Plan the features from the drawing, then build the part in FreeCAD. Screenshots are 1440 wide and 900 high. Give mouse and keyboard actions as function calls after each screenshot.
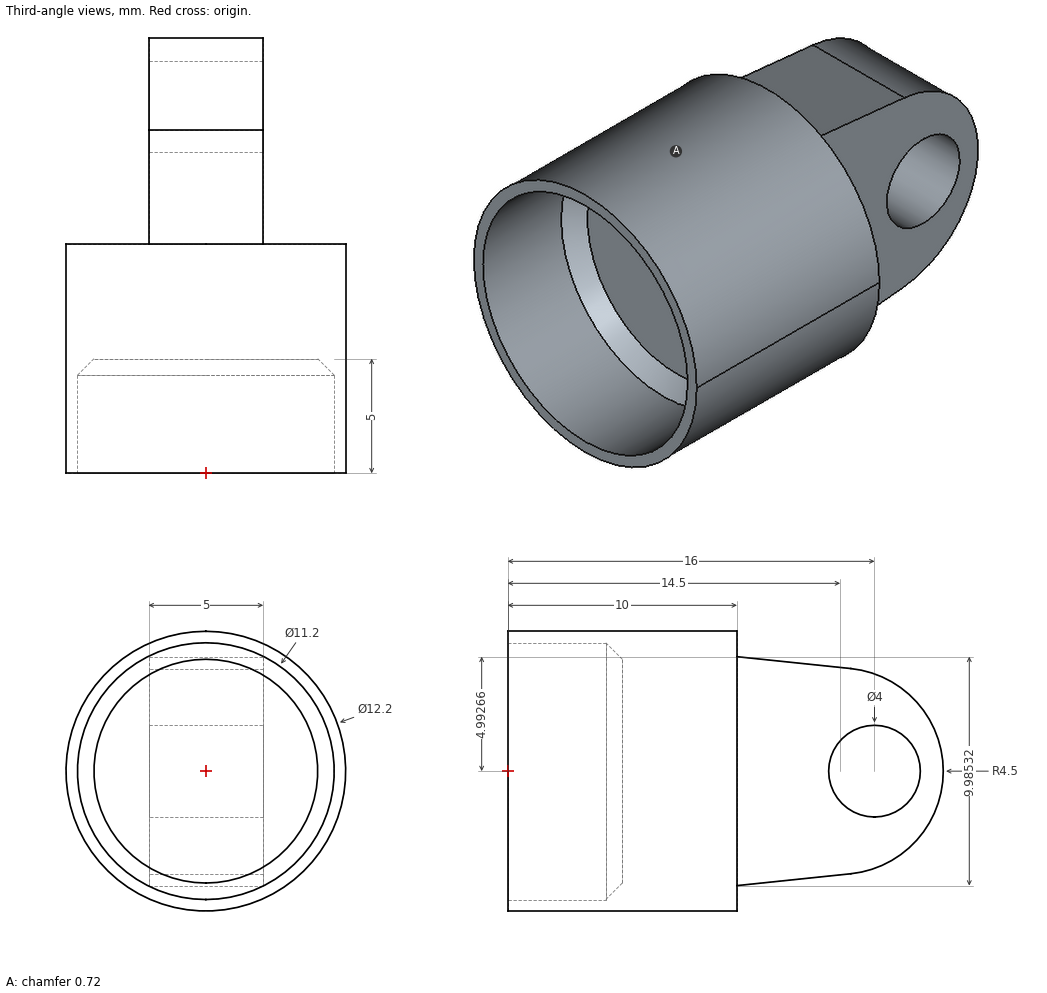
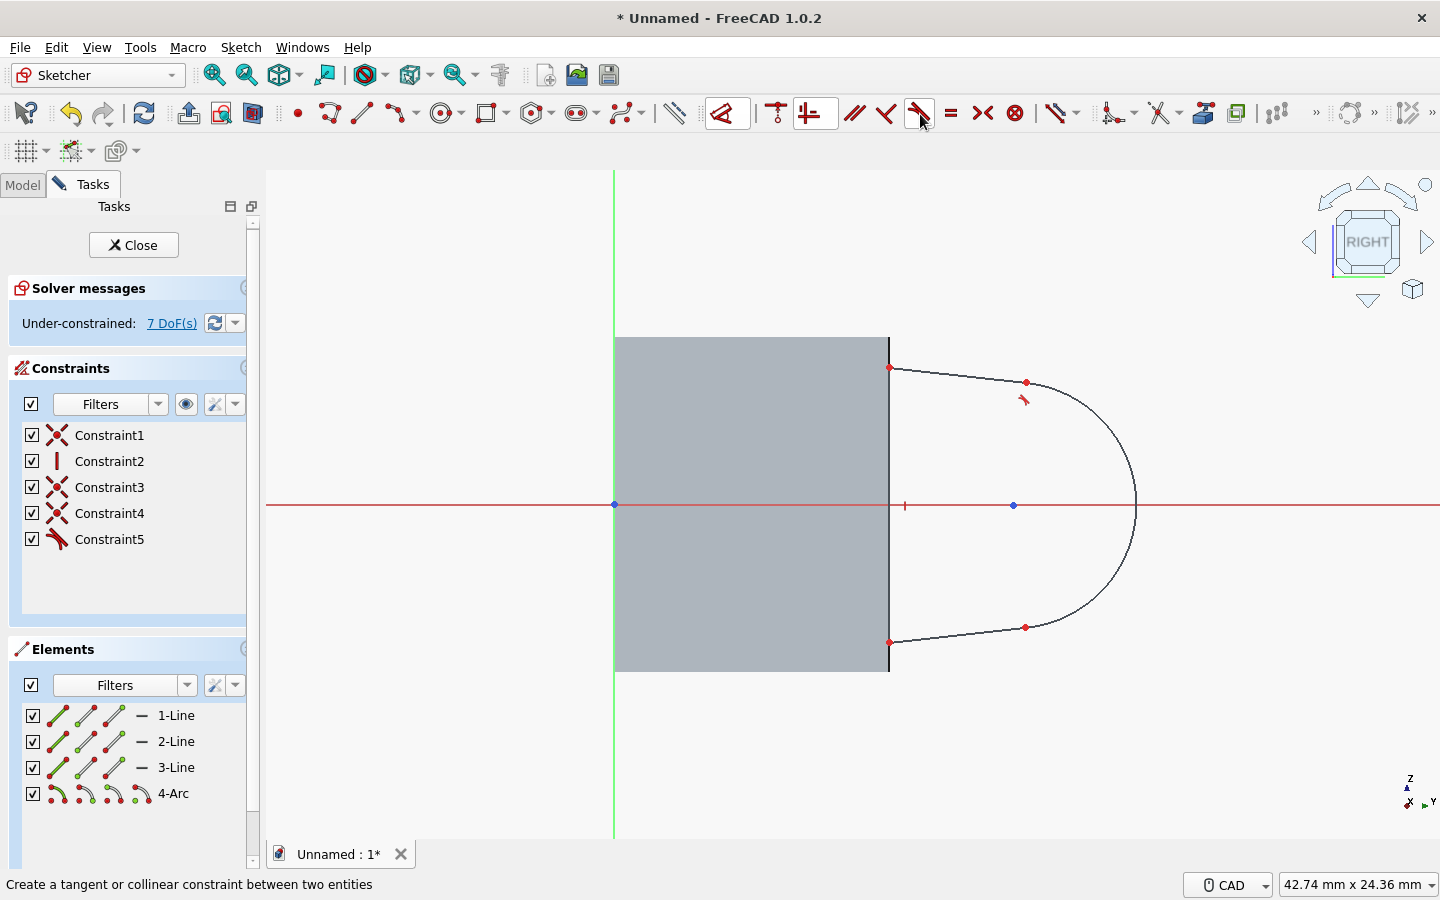
click(930, 639)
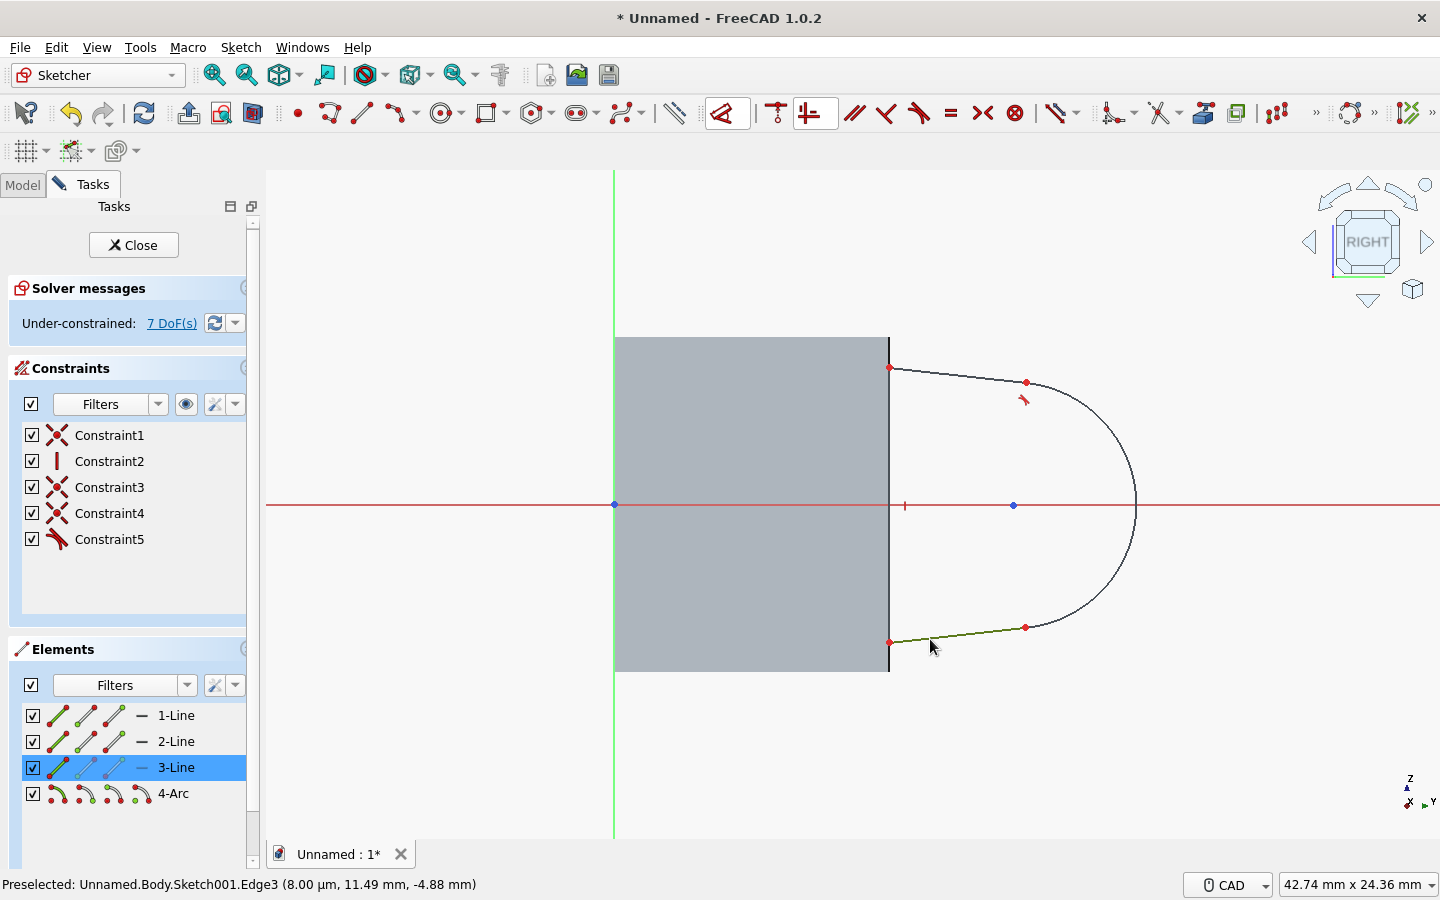
click(1115, 574)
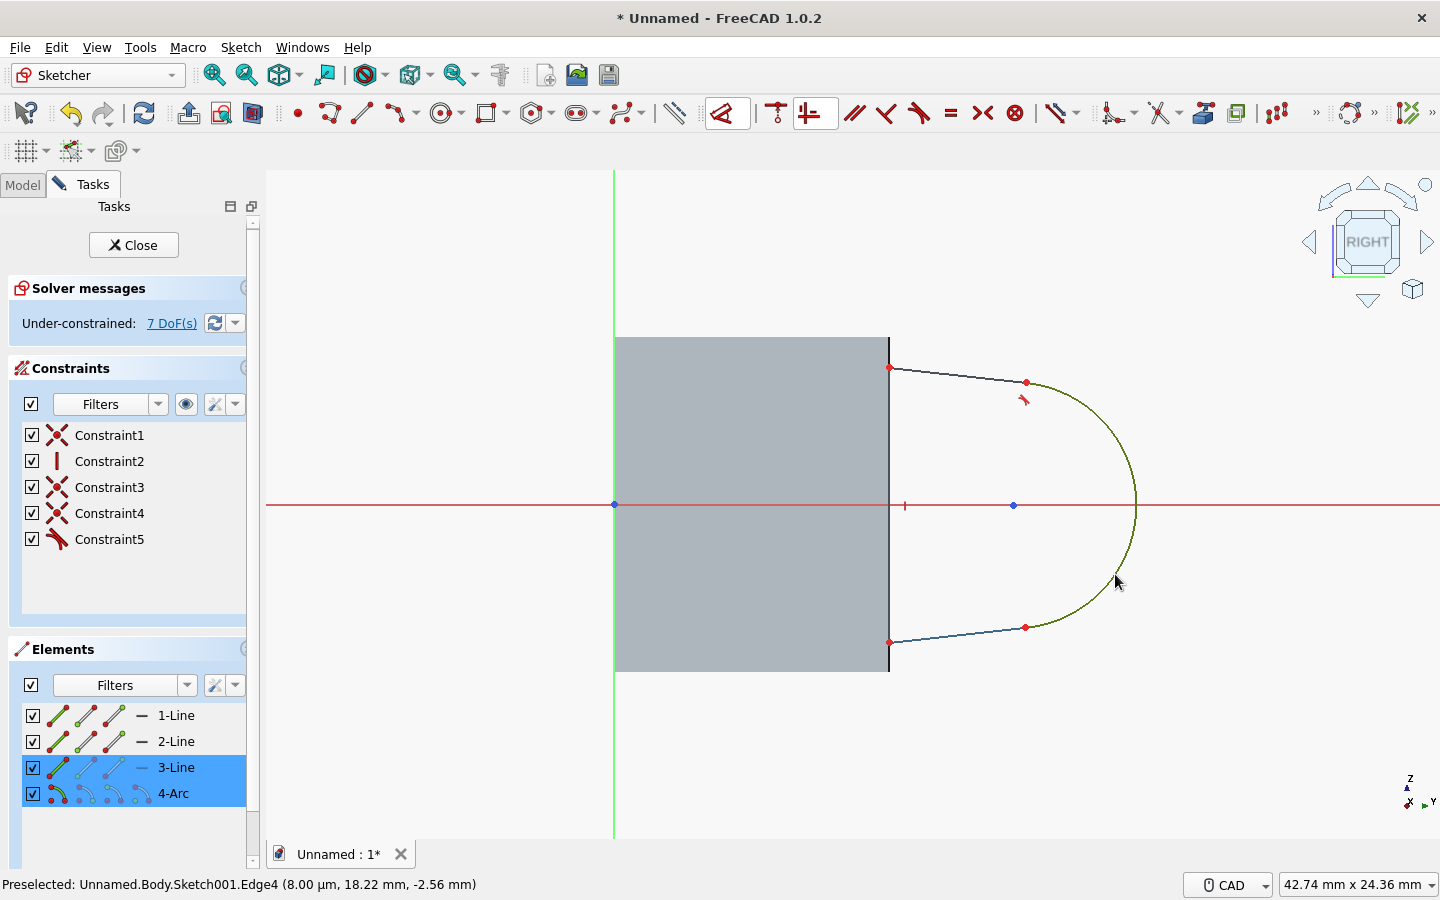
key(t)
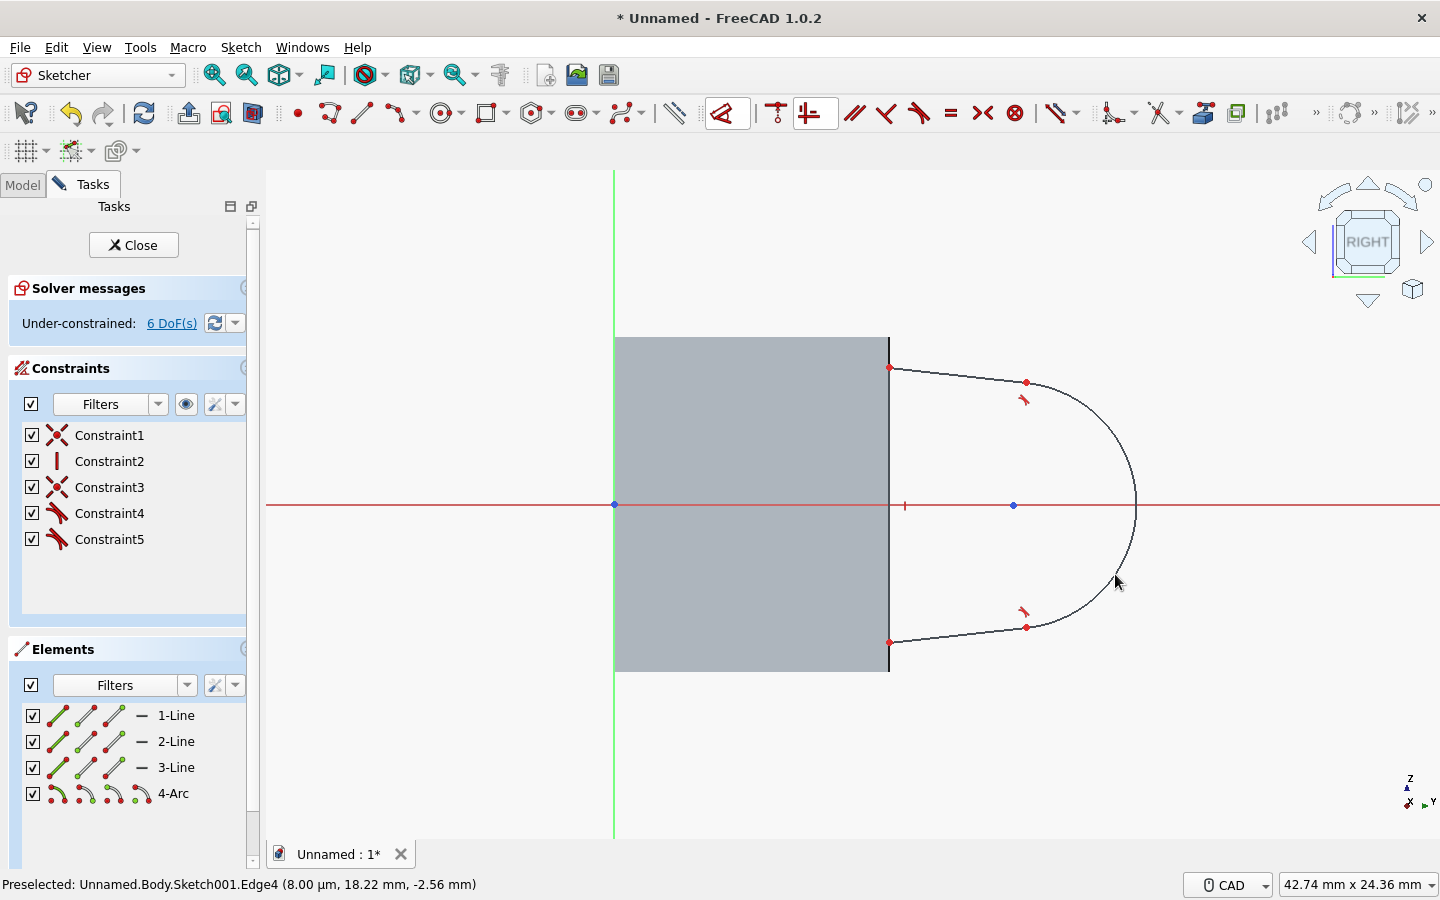
click(1013, 506)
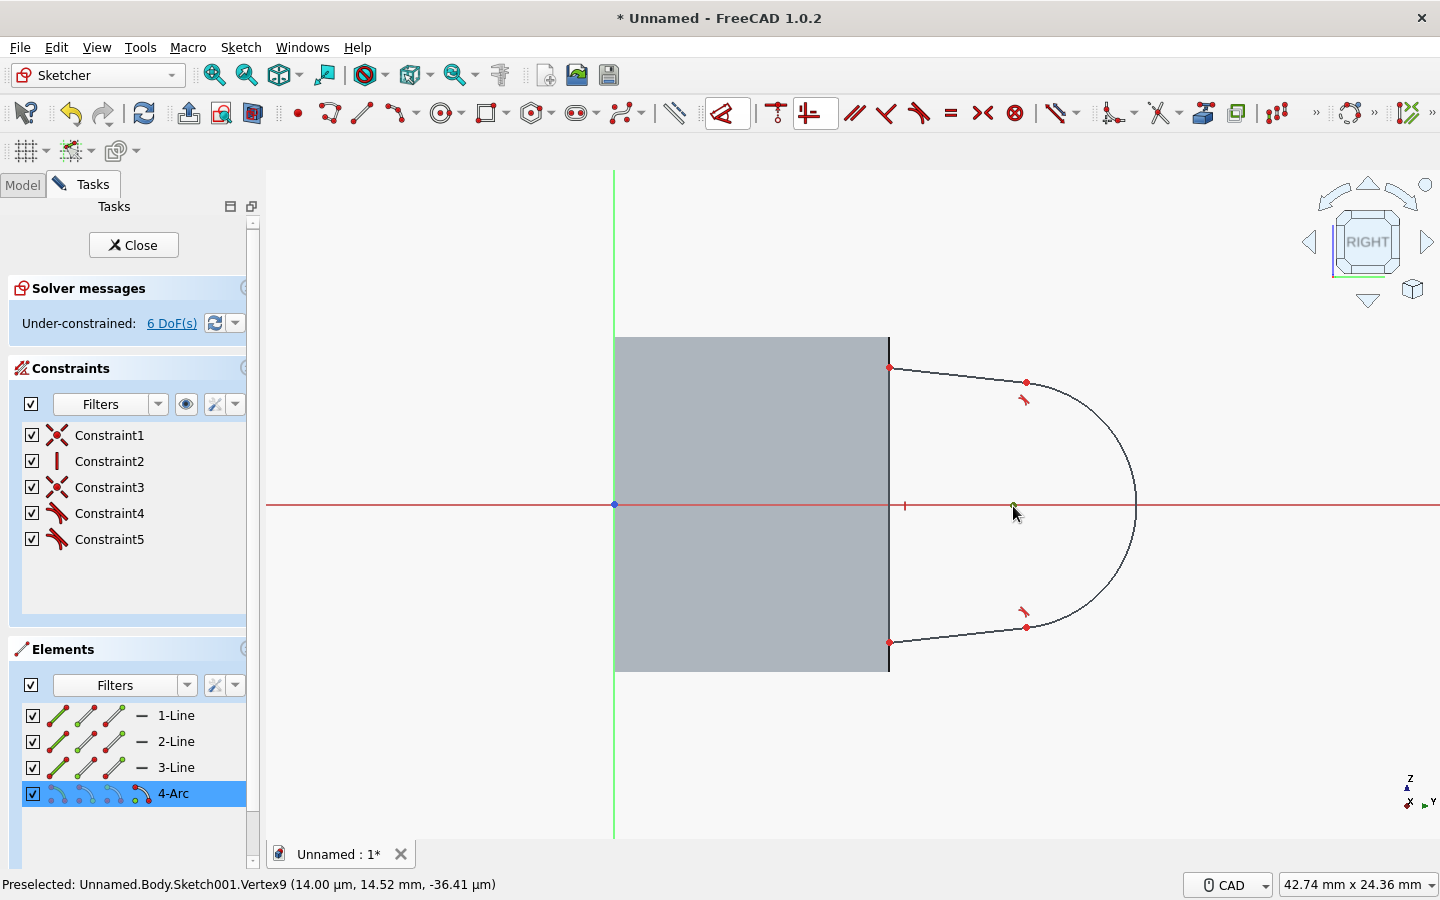
click(364, 505)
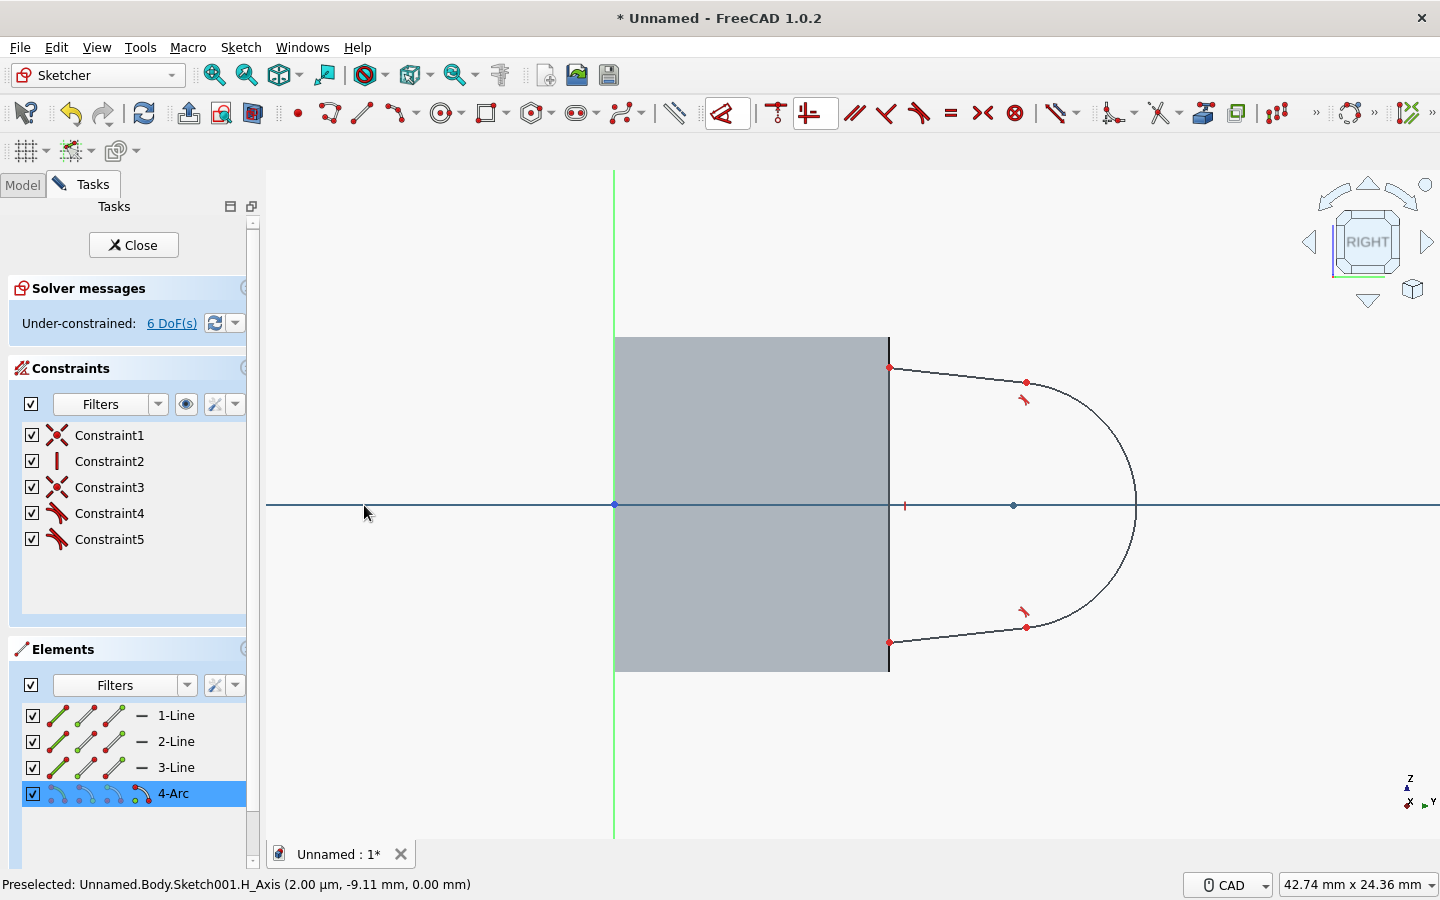
key(c)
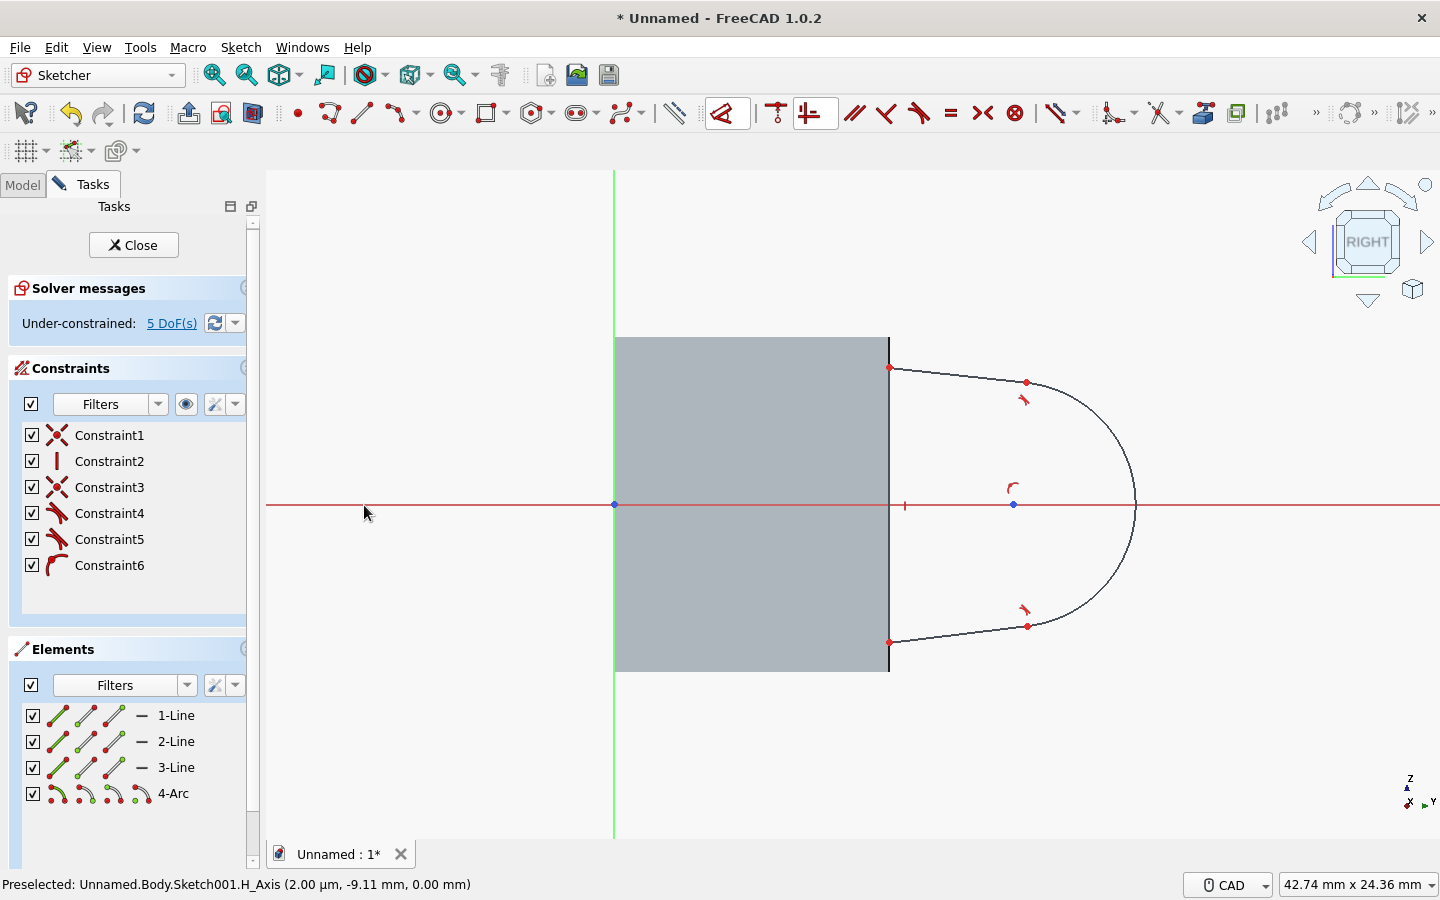
key(d)